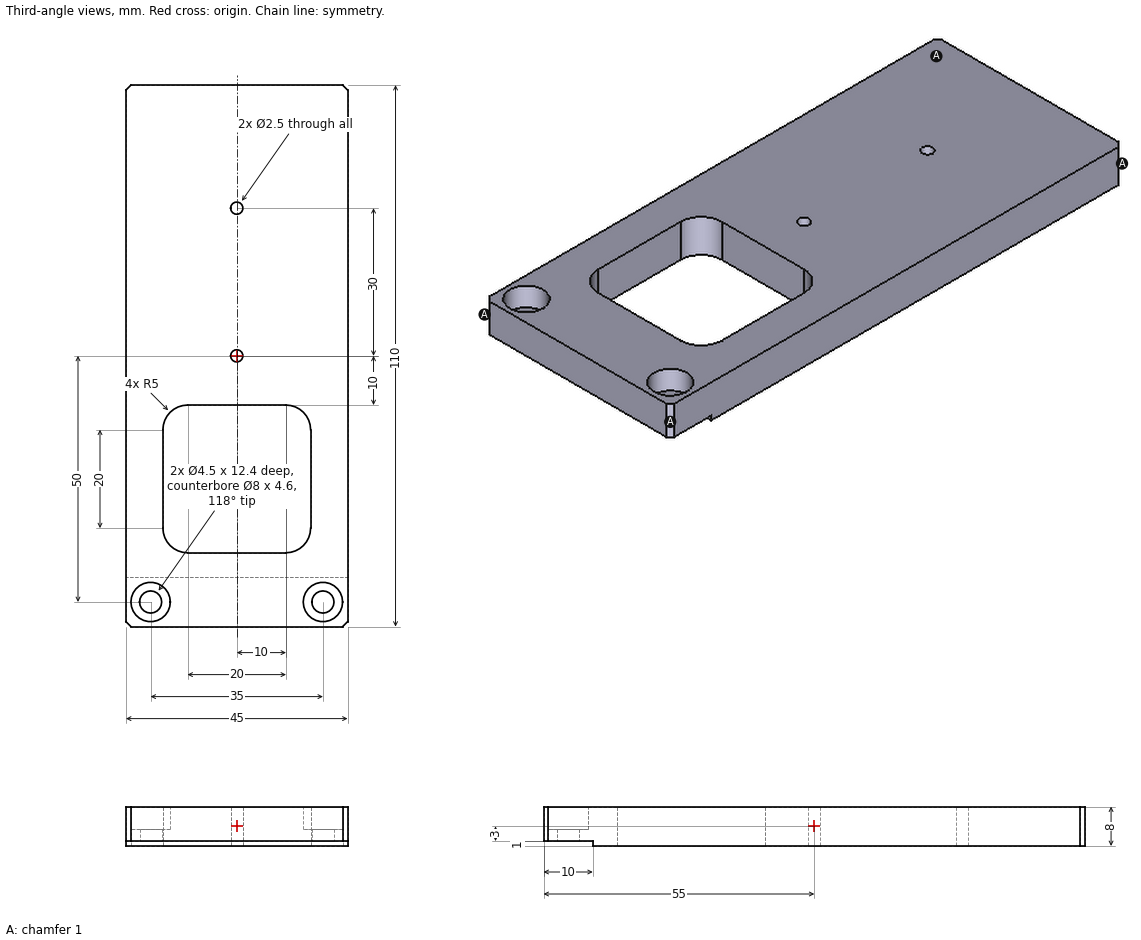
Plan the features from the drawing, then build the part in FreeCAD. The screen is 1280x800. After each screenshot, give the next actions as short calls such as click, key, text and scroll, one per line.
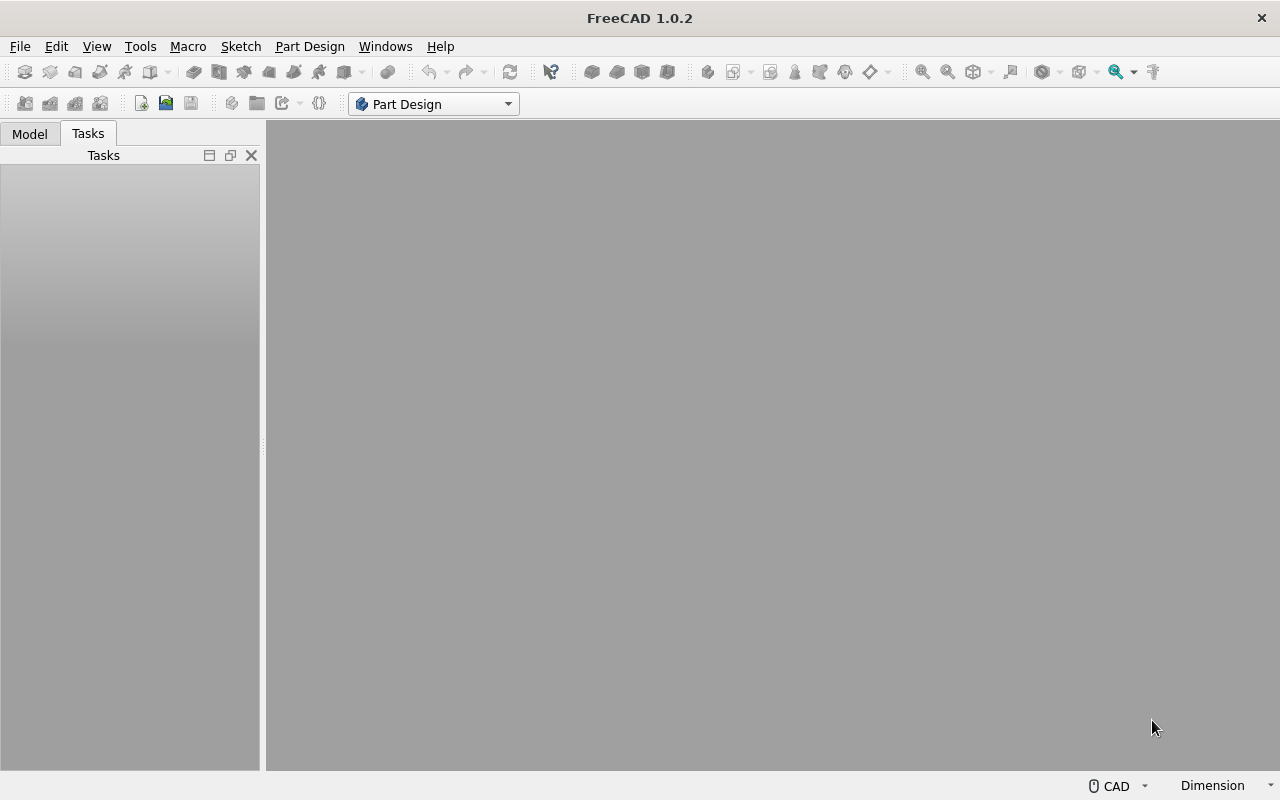
click(141, 104)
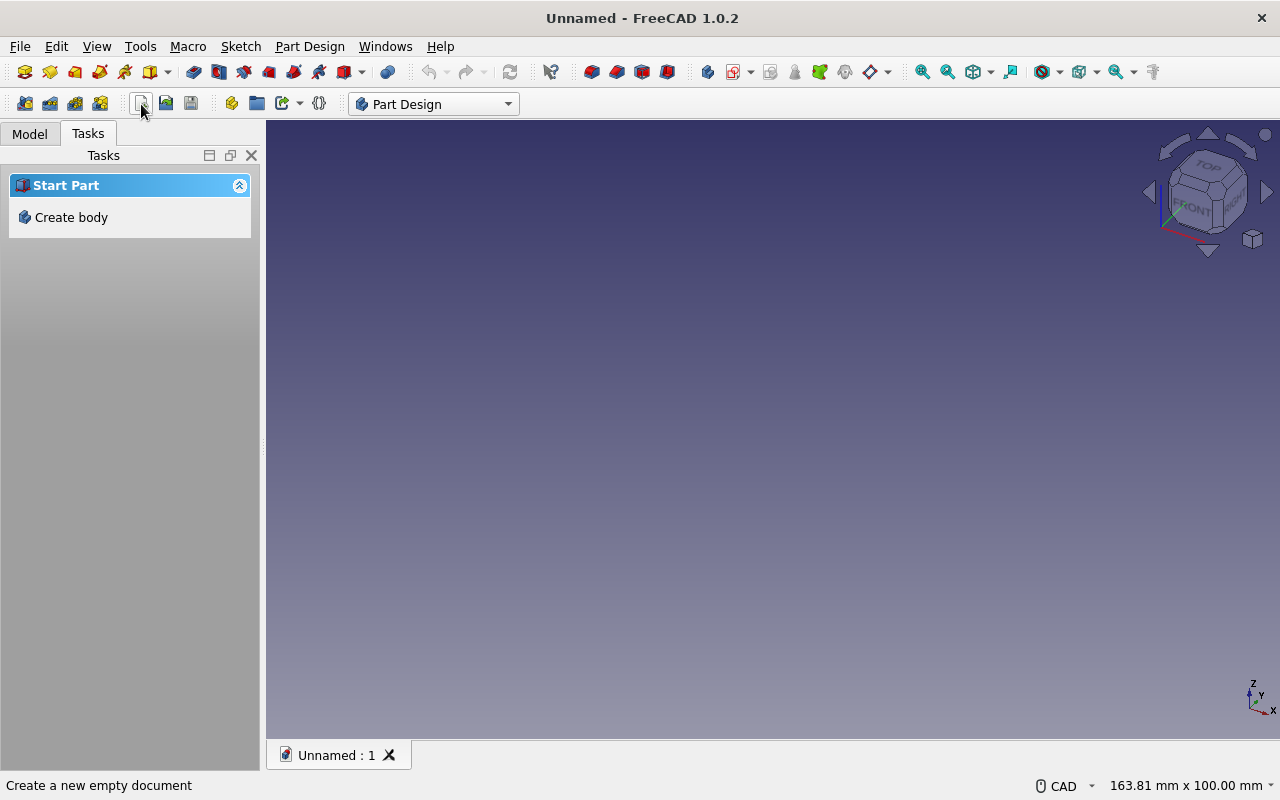
click(732, 72)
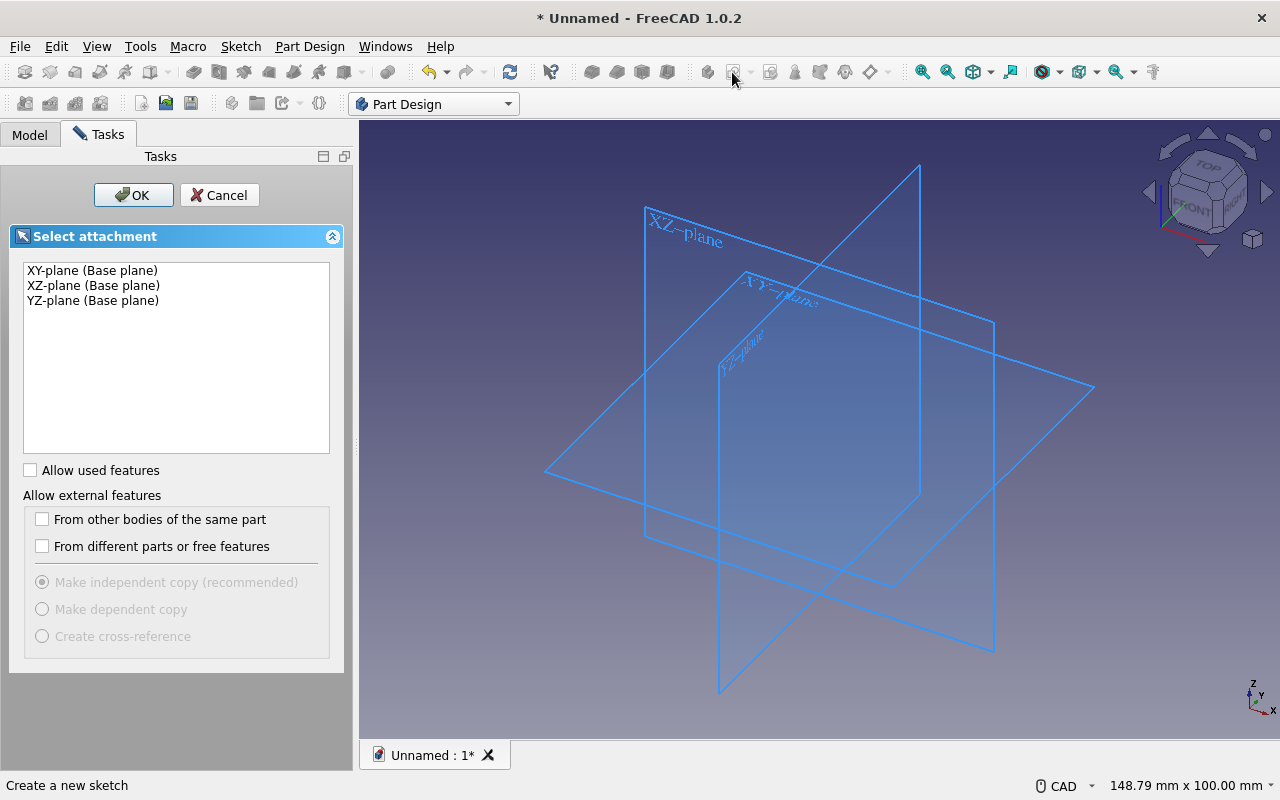
click(84, 270)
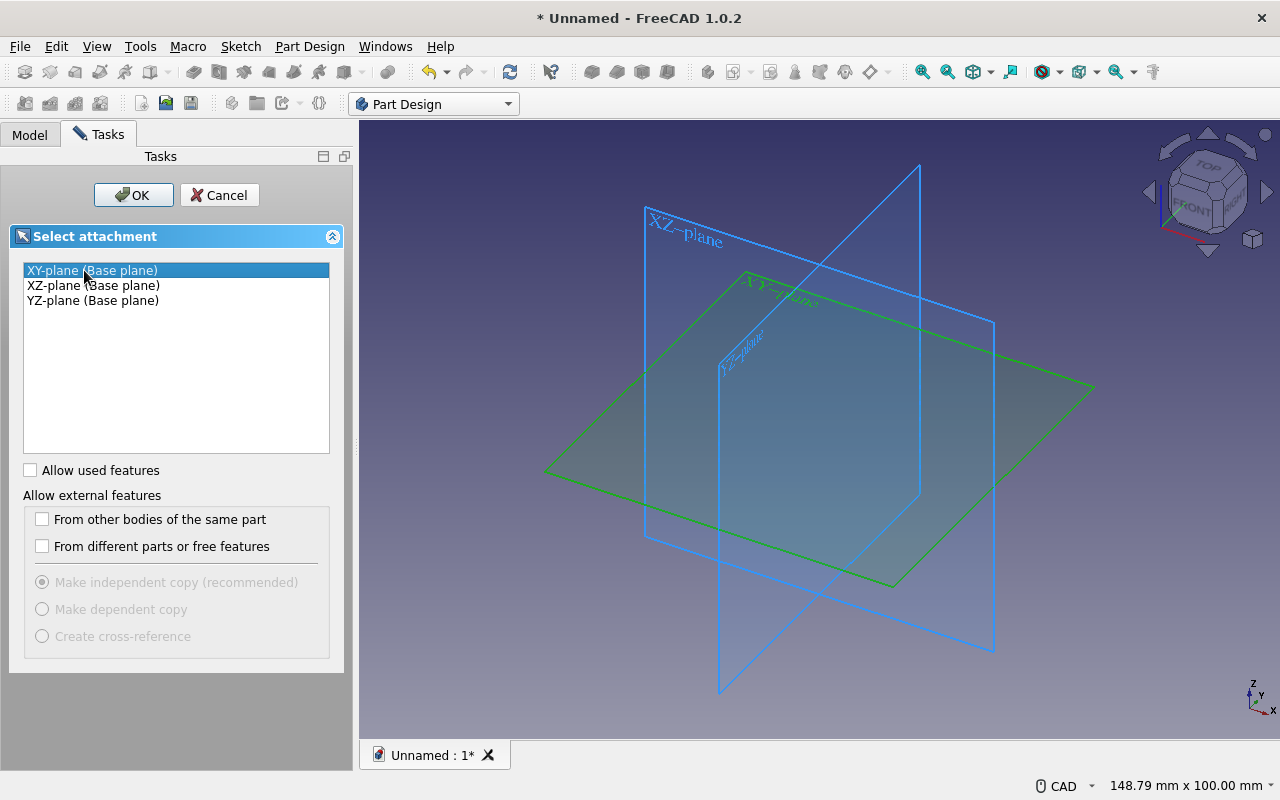
click(134, 195)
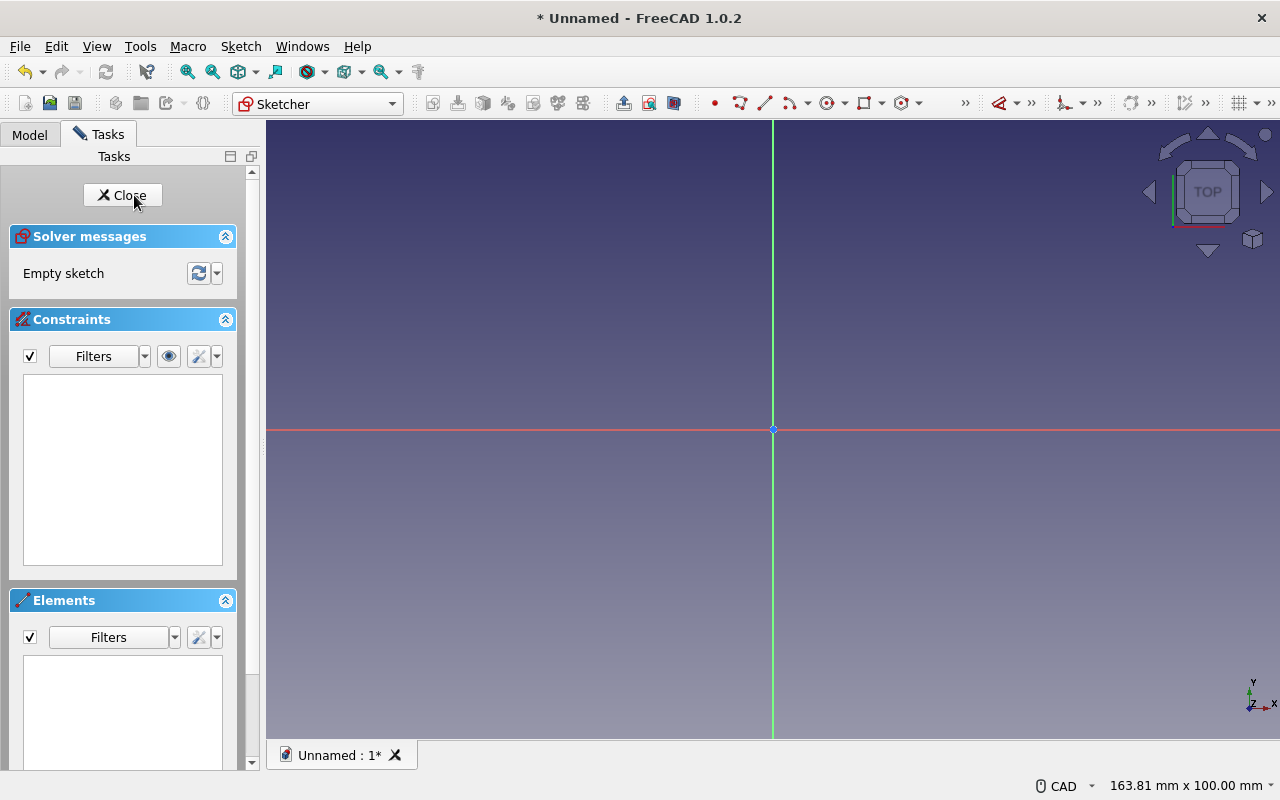
scroll(621, 430, down, 3)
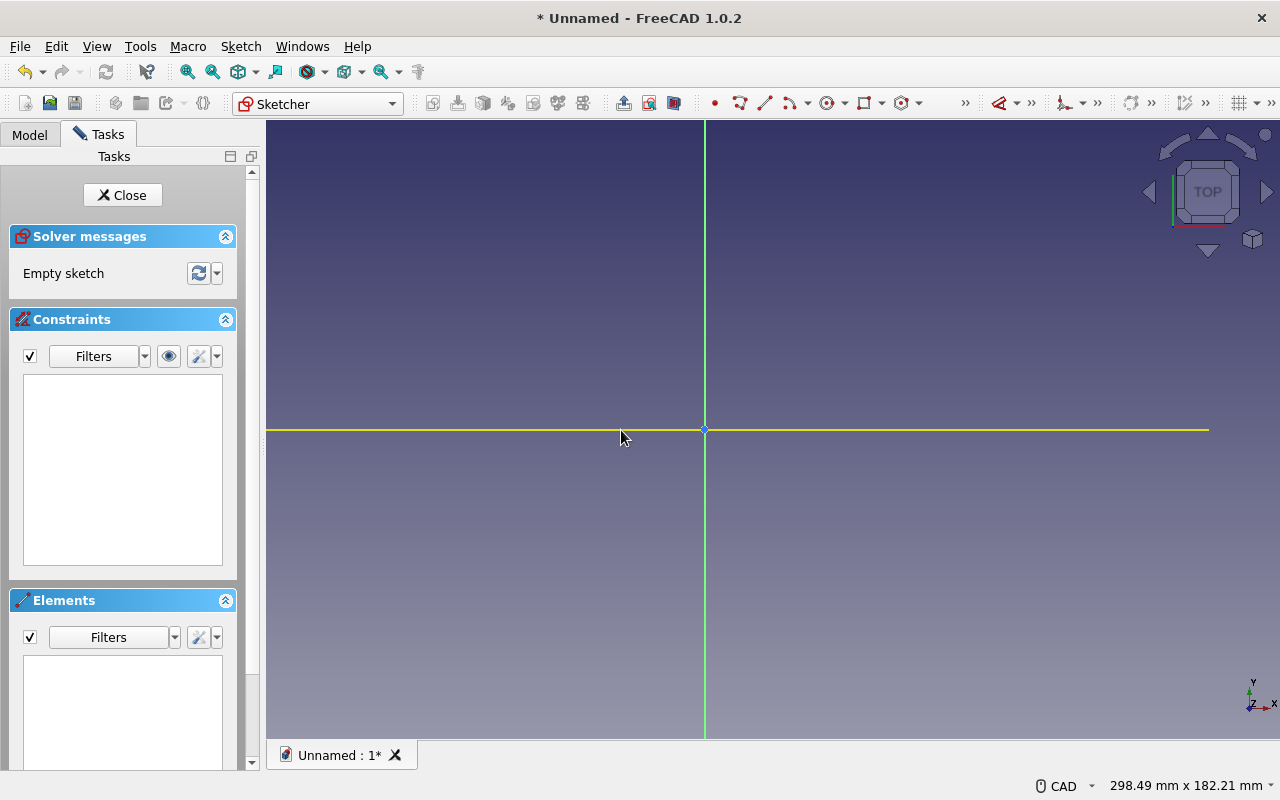
click(882, 104)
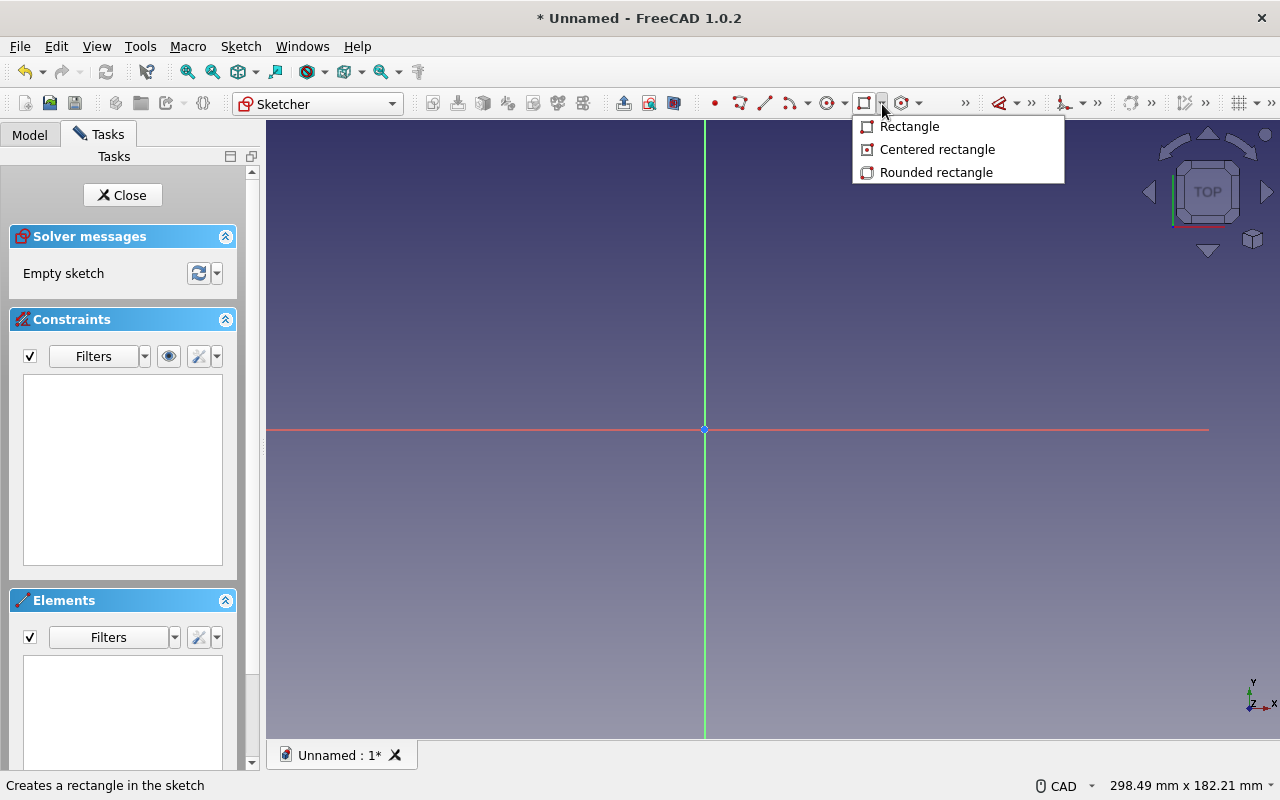
click(958, 150)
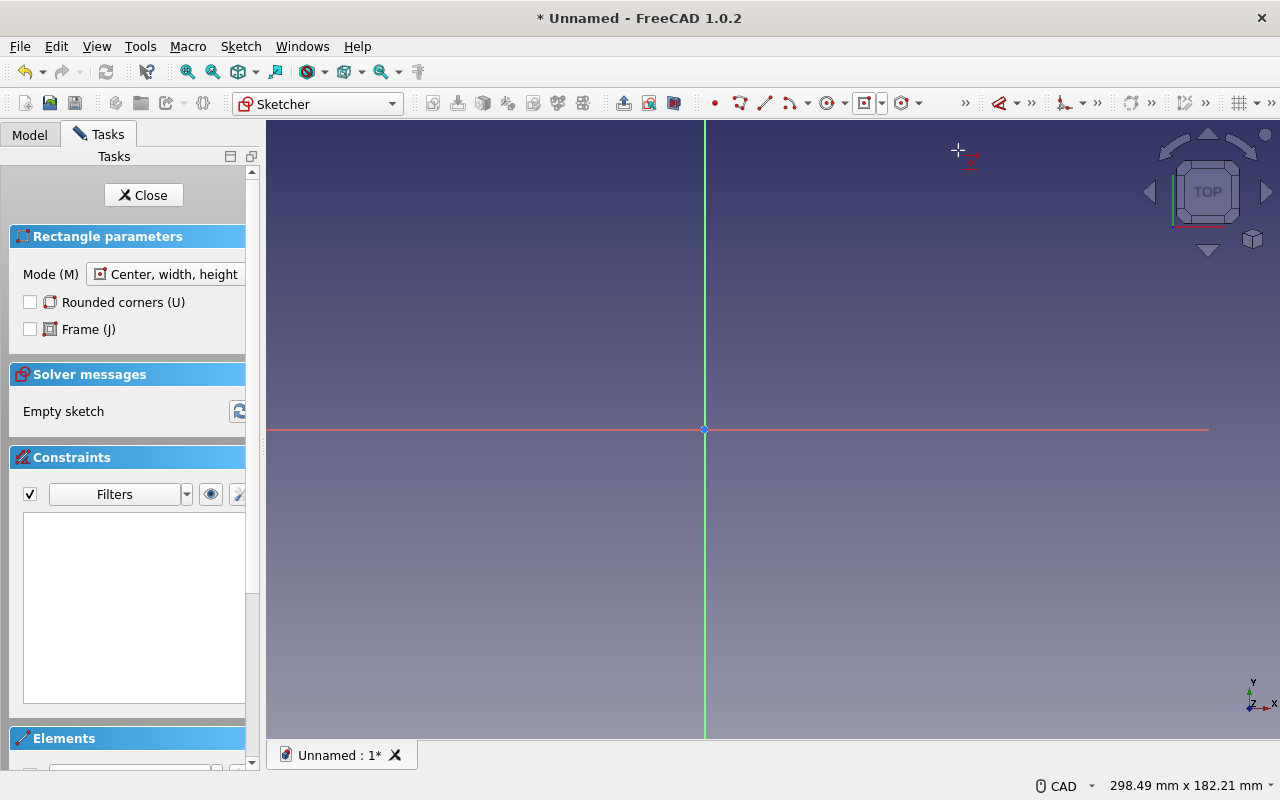
click(705, 430)
move(781, 243)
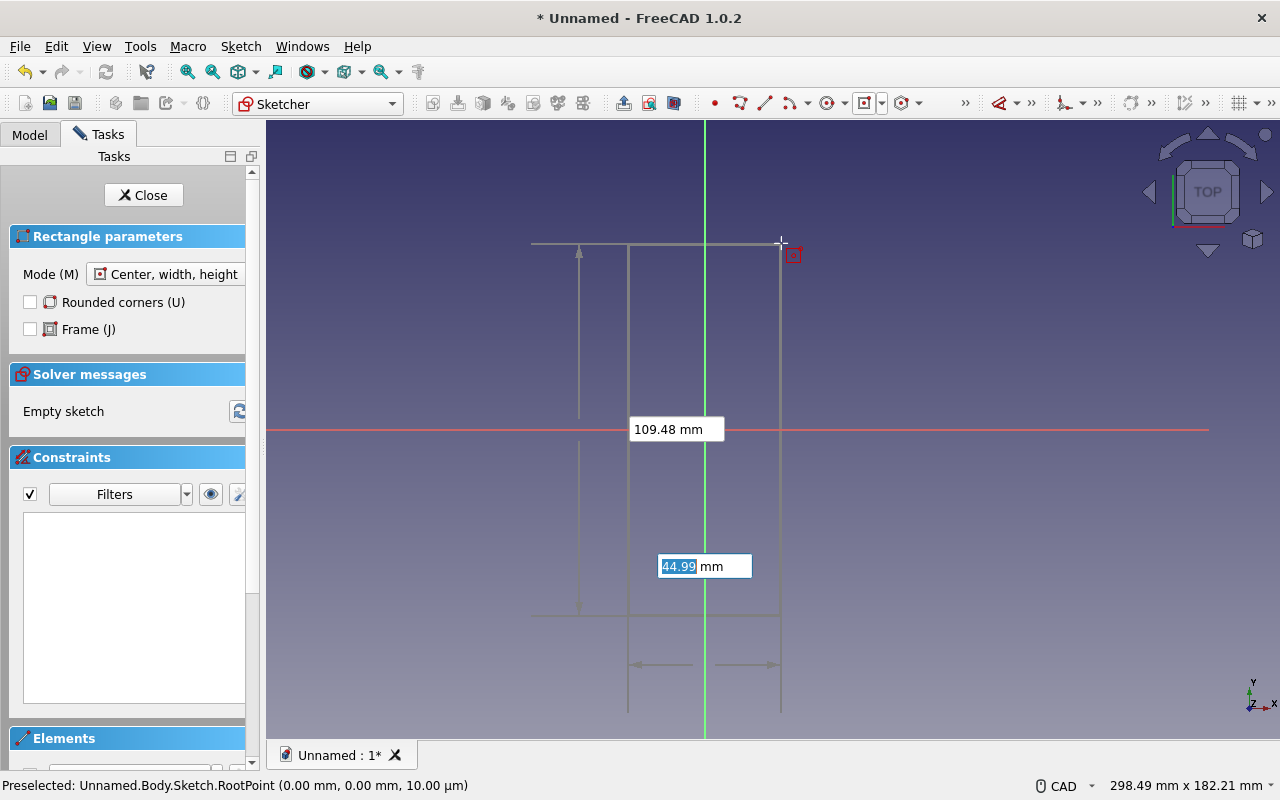
text(45)
key(Tab)
text(110)
key(Return)
key(Escape)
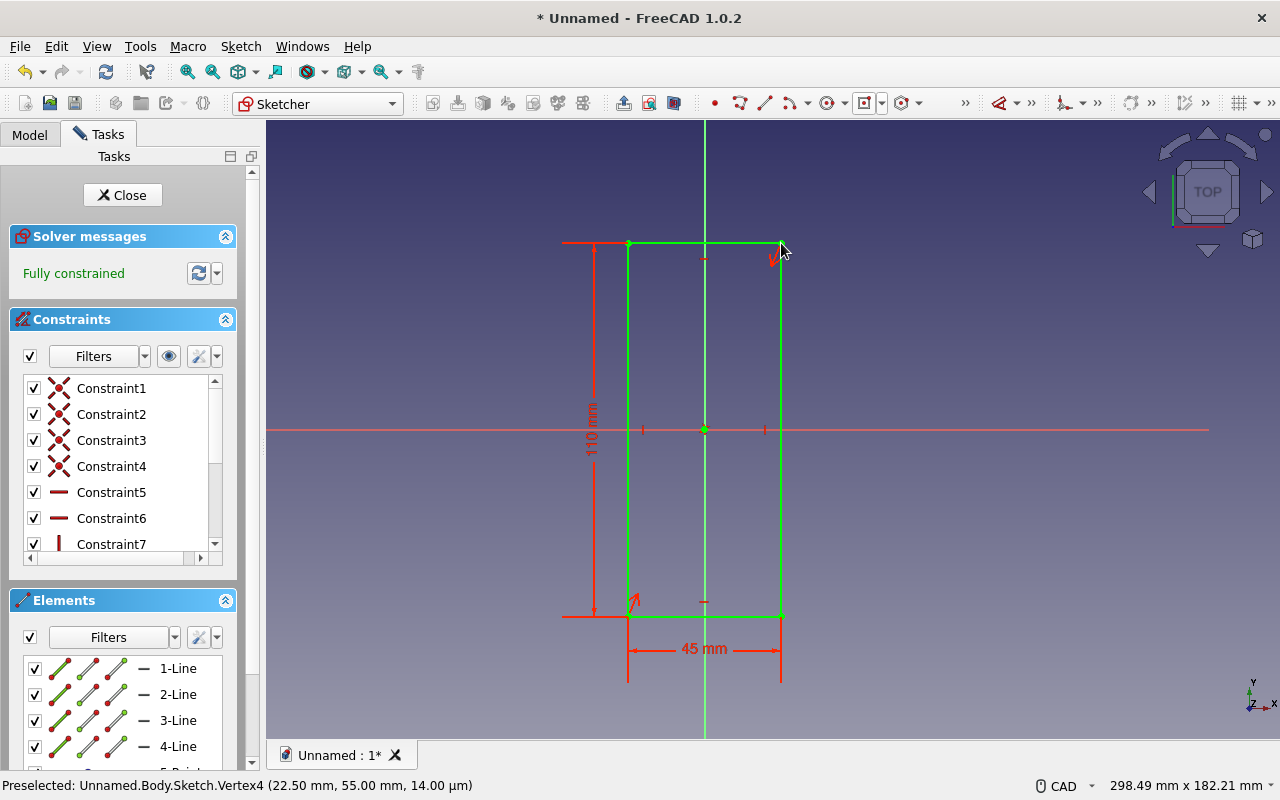
click(123, 195)